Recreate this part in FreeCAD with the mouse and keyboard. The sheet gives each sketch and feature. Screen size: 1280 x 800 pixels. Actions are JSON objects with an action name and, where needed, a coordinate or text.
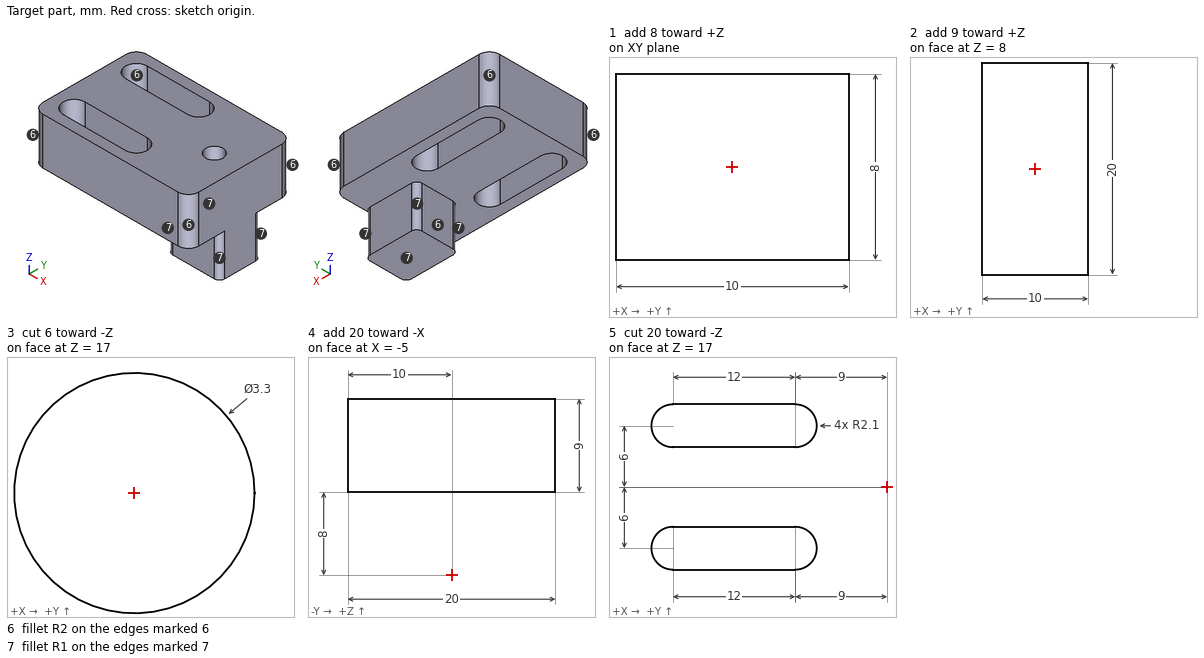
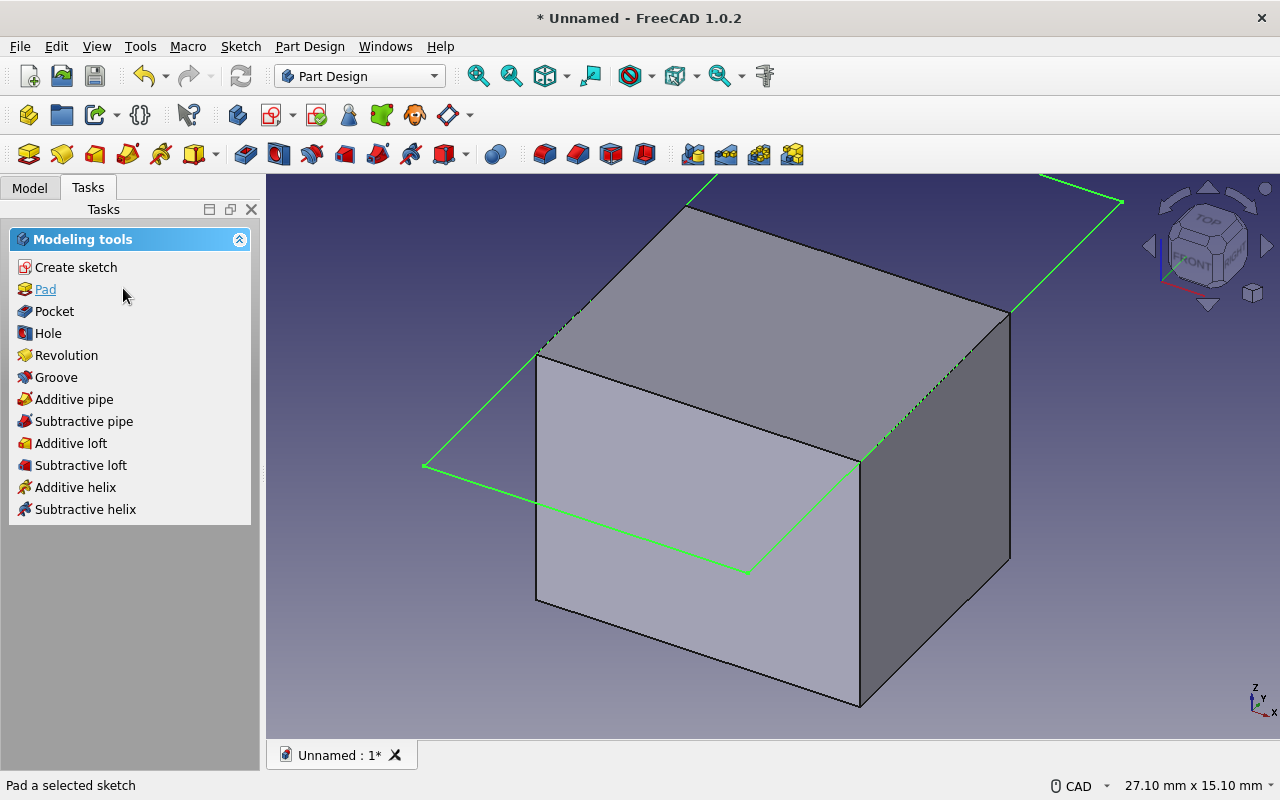
{"action": "left_click", "coordinate": [29, 154]}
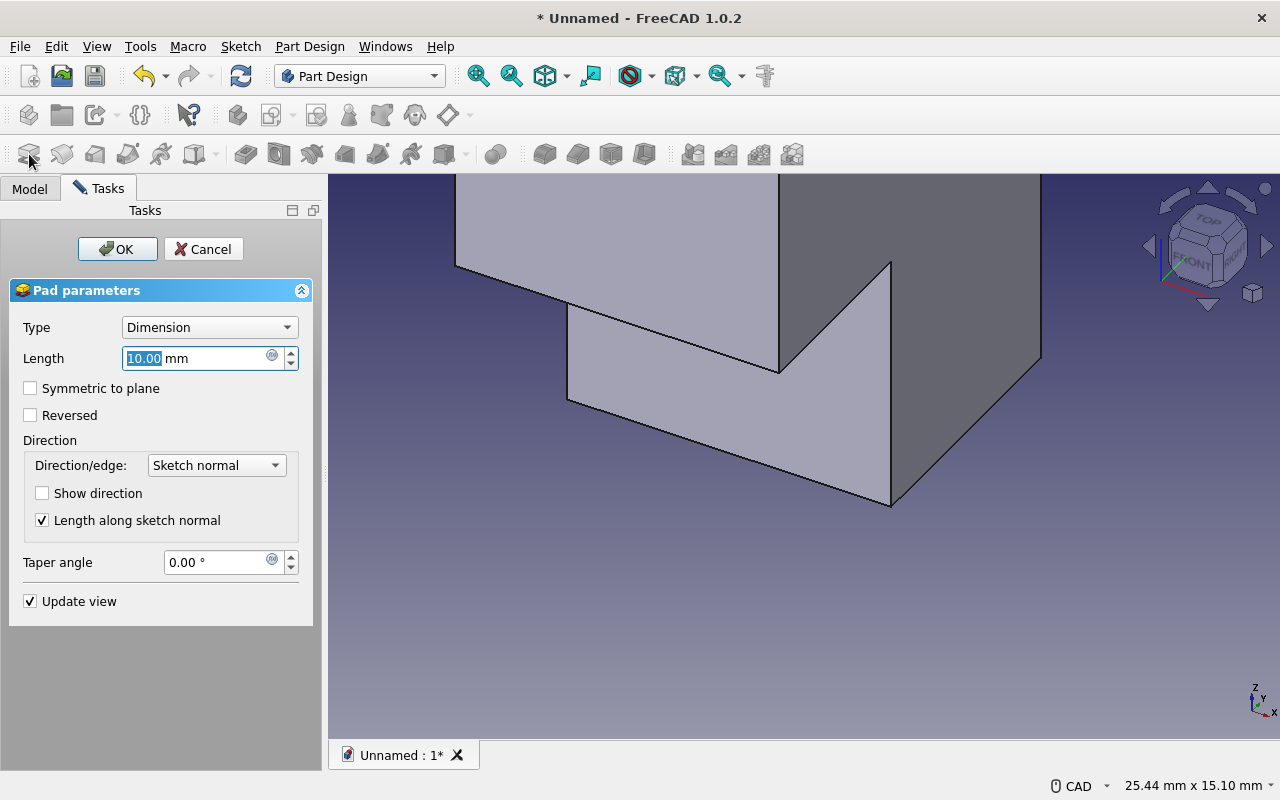
{"action": "type", "text": "9"}
{"action": "key", "text": "Tab"}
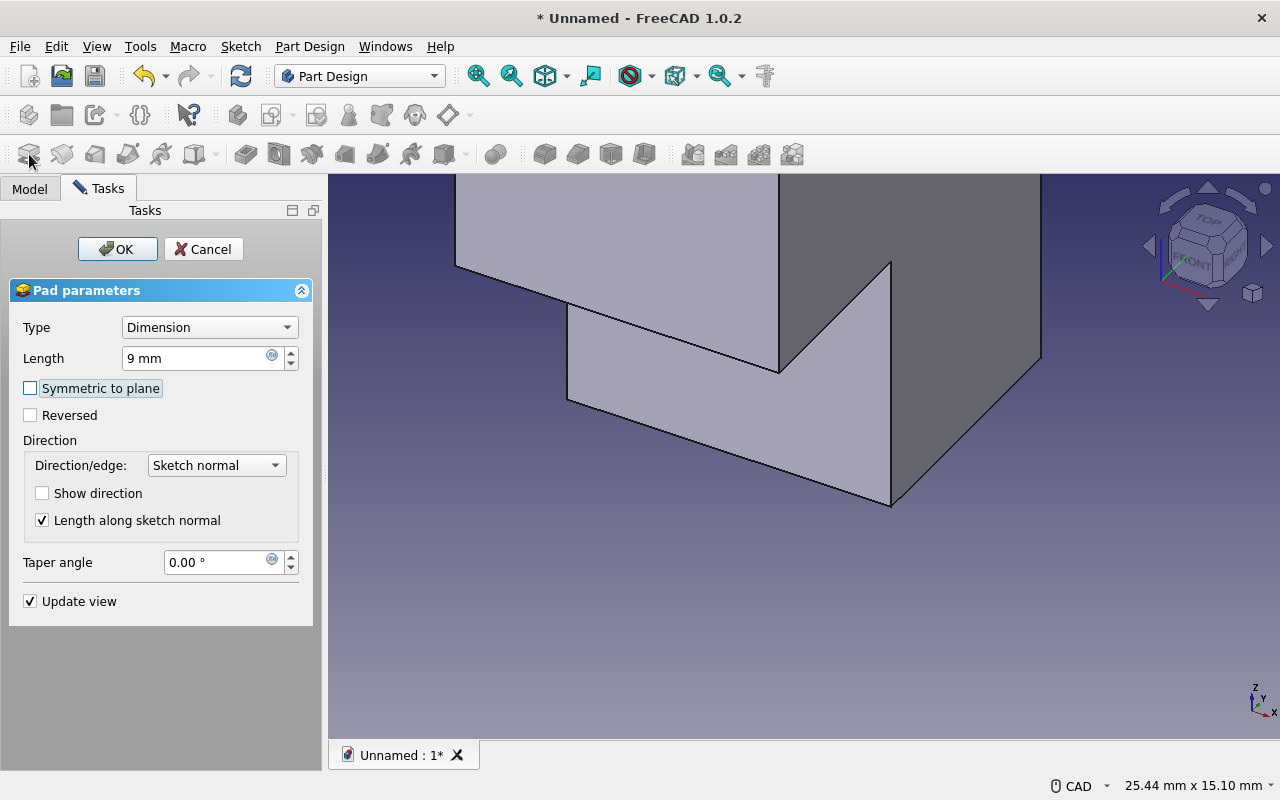
{"action": "left_click", "coordinate": [118, 249]}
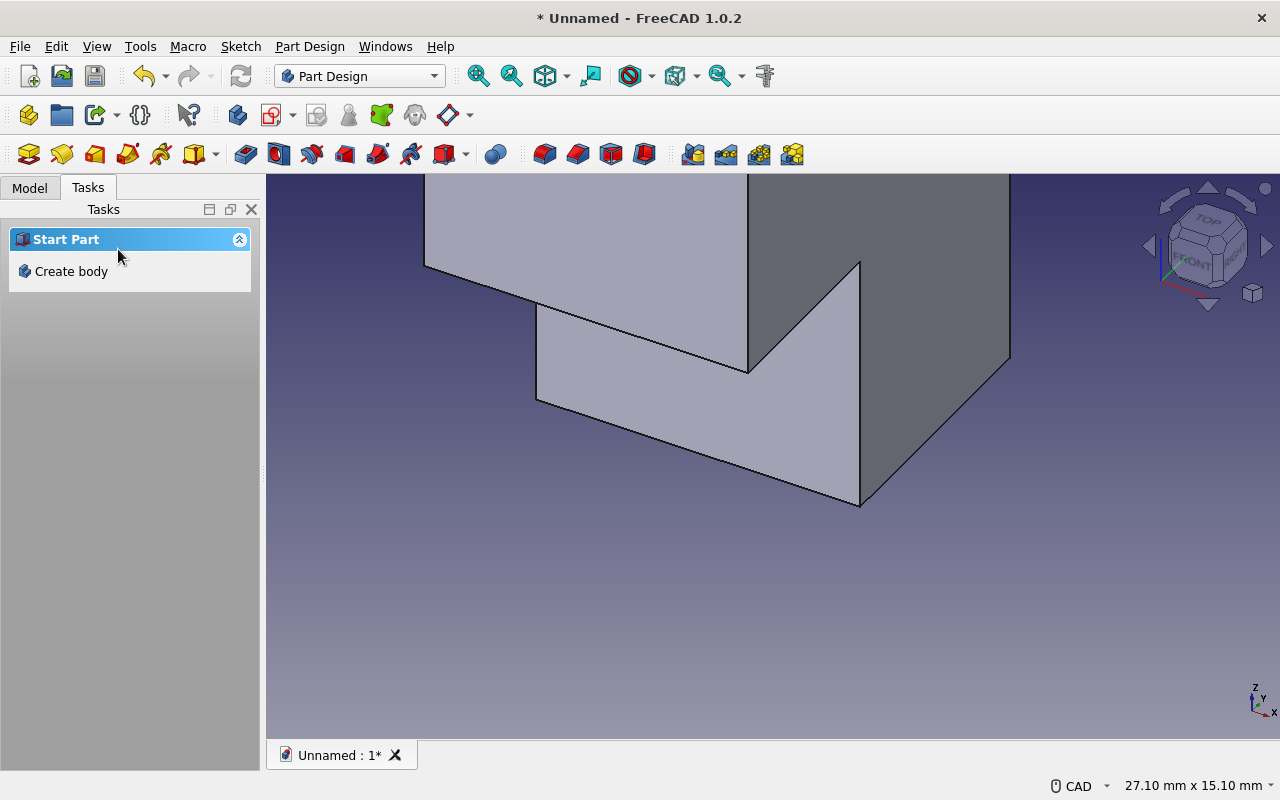
{"action": "left_click", "coordinate": [479, 76]}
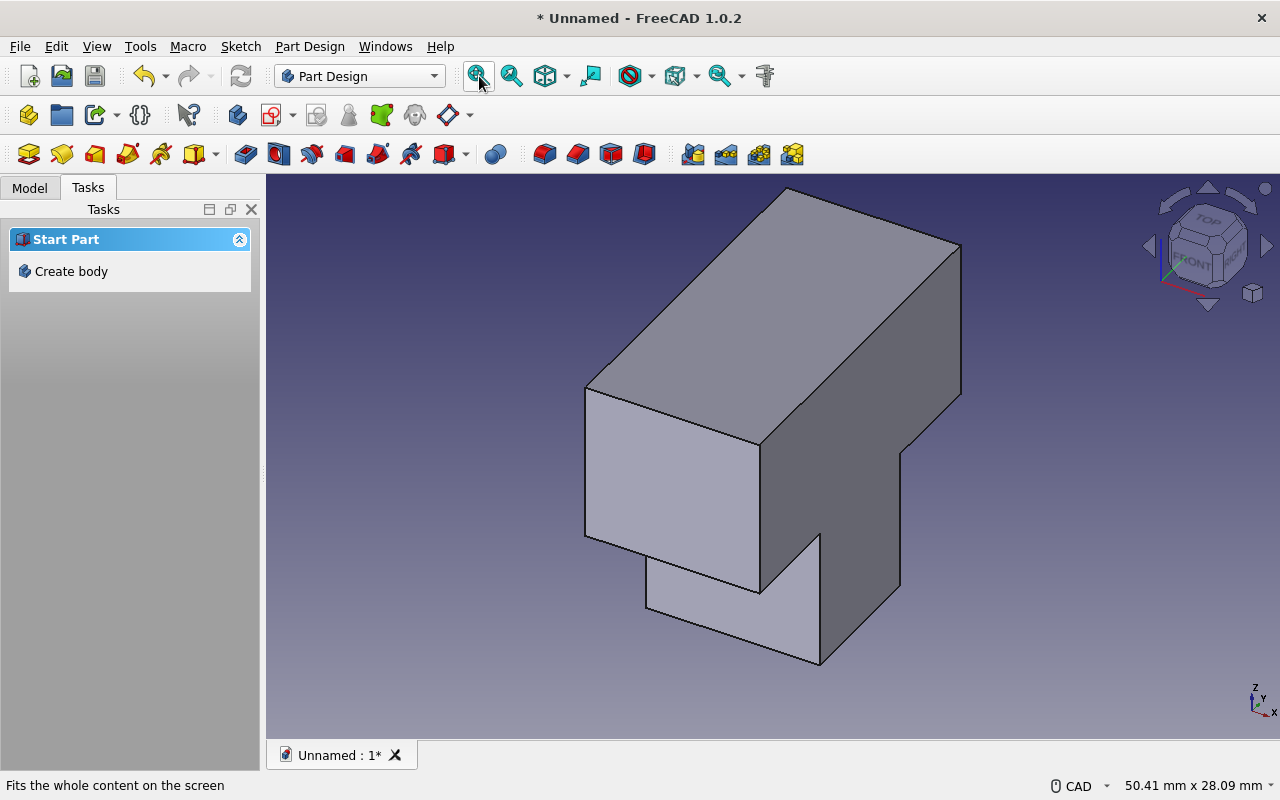
{"action": "left_click", "coordinate": [802, 287]}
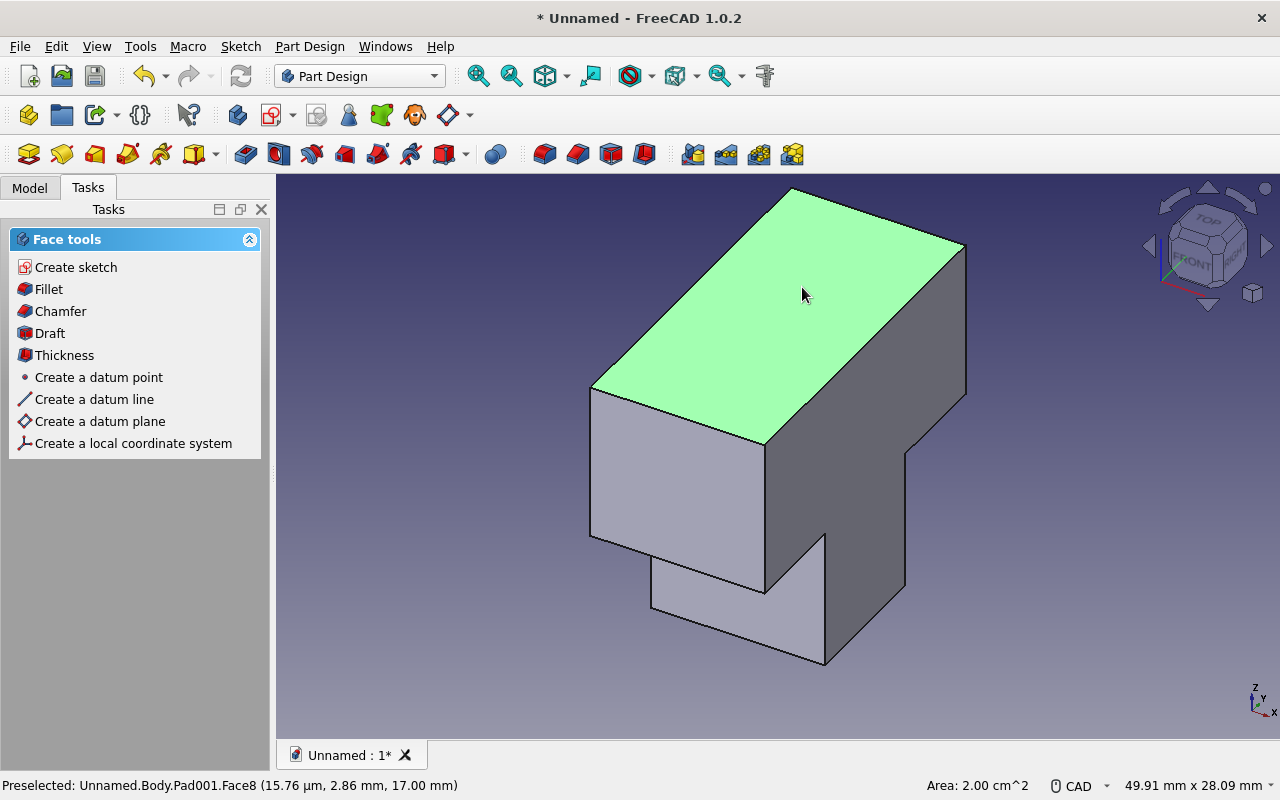
{"action": "left_click", "coordinate": [270, 116]}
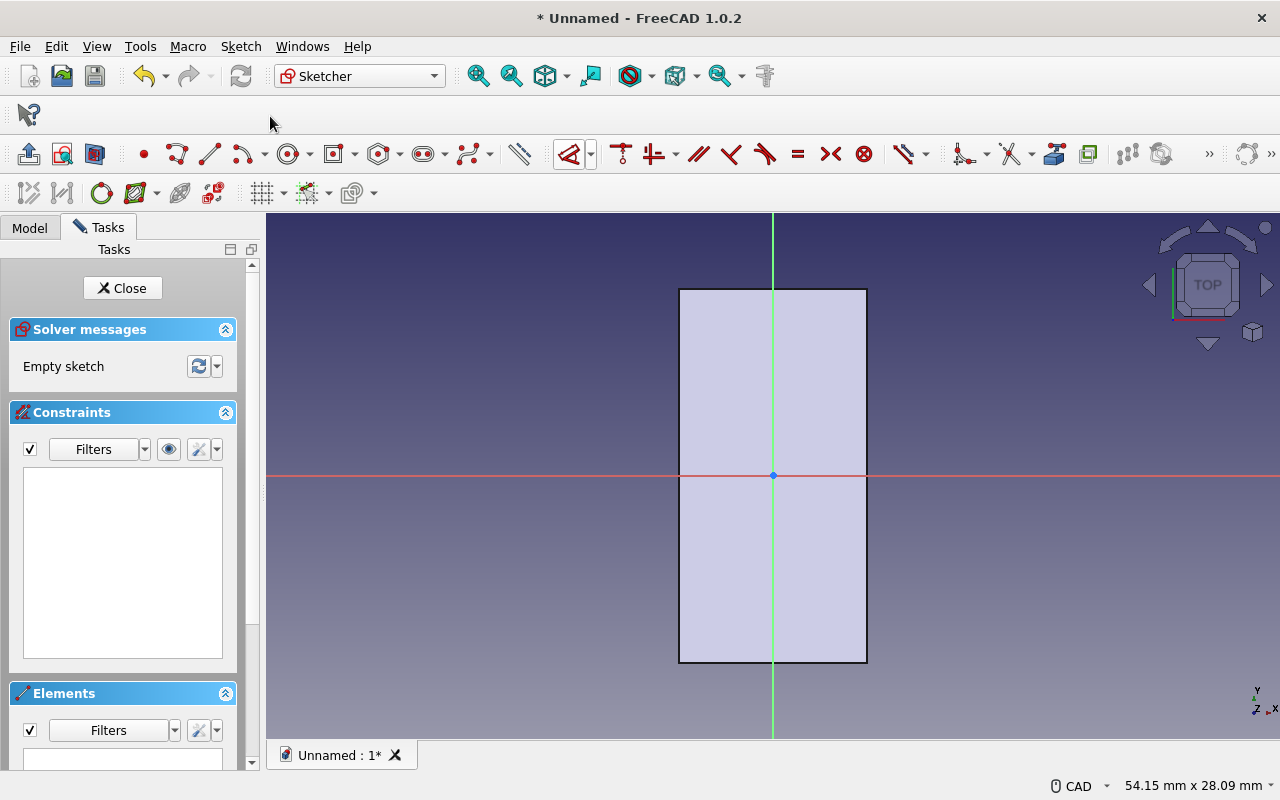
{"action": "scroll", "coordinate": [790, 476], "scroll_direction": "up", "scroll_amount": 8}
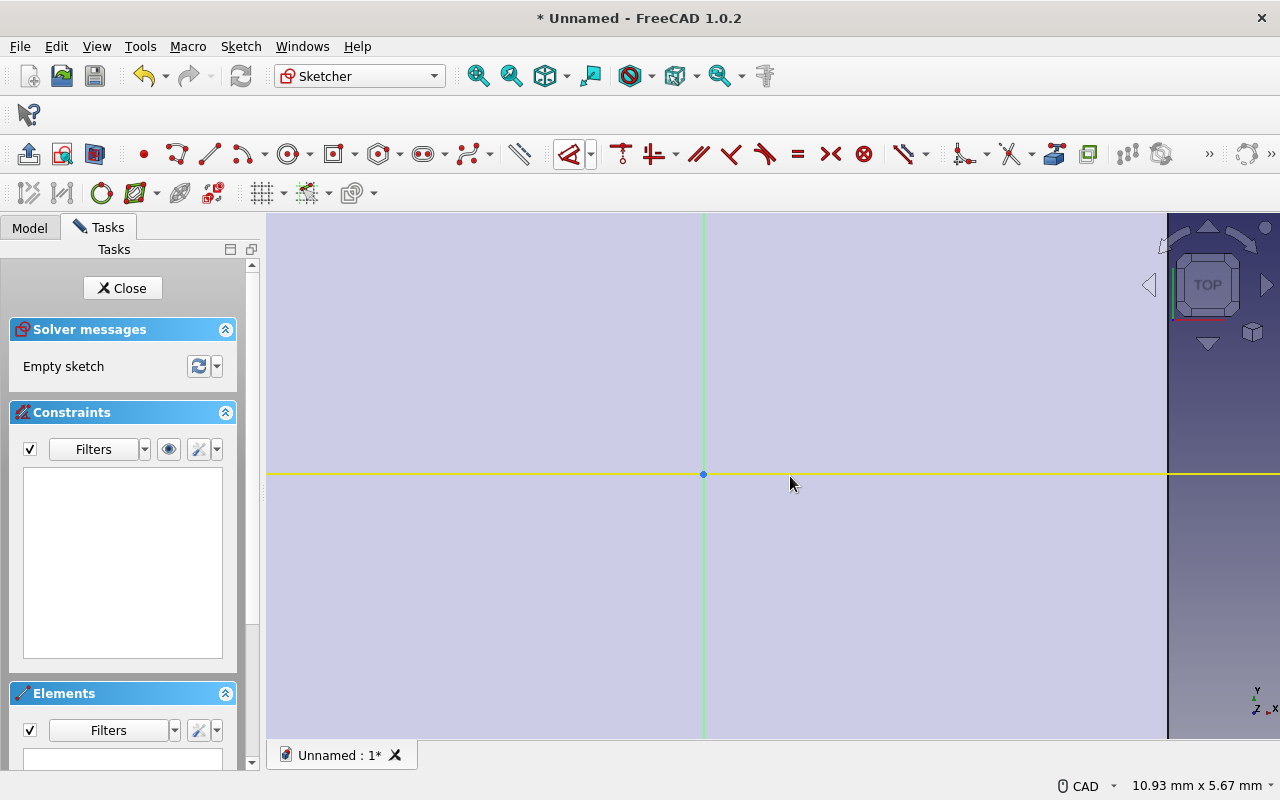
{"action": "left_click", "coordinate": [288, 154]}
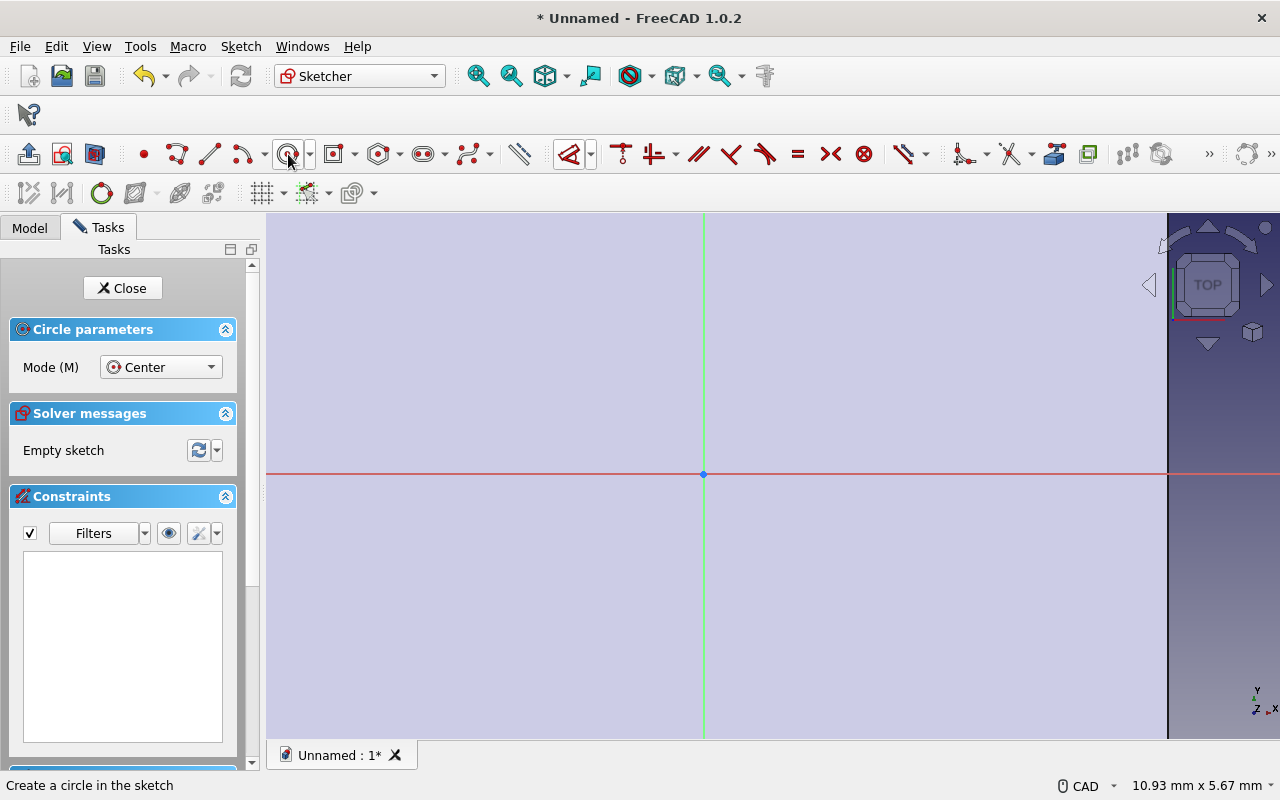
{"action": "left_click", "coordinate": [704, 474]}
{"action": "mouse_move", "coordinate": [812, 366]}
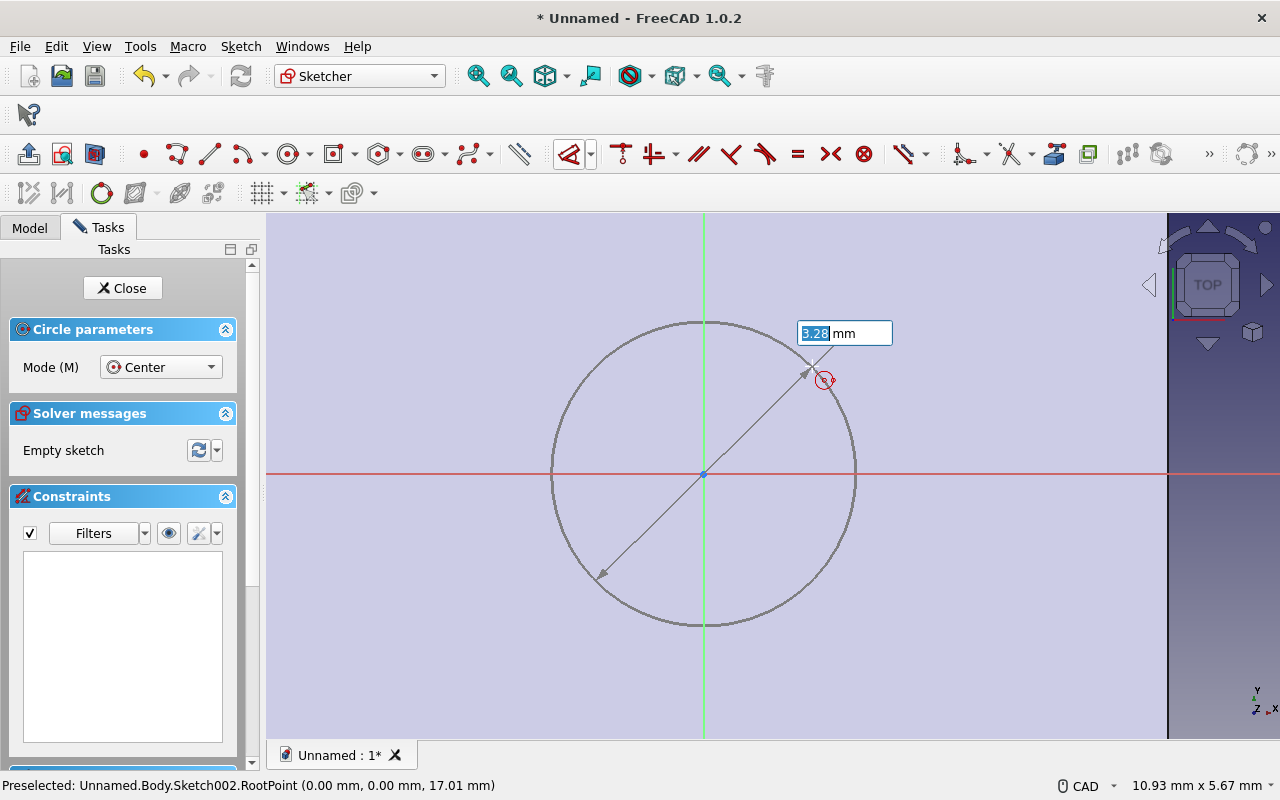
{"action": "type", "text": "3.3"}
{"action": "key", "text": "Return"}
{"action": "key", "text": "Escape"}